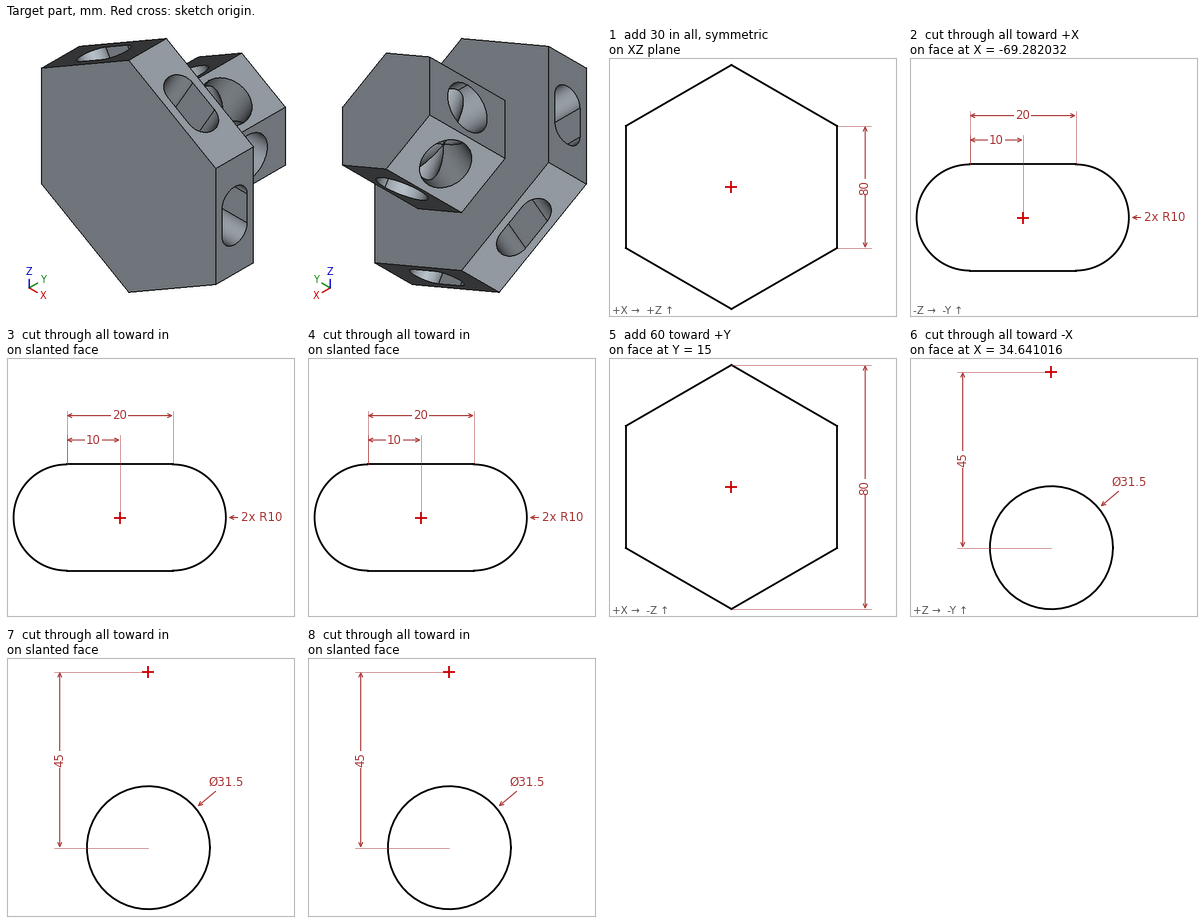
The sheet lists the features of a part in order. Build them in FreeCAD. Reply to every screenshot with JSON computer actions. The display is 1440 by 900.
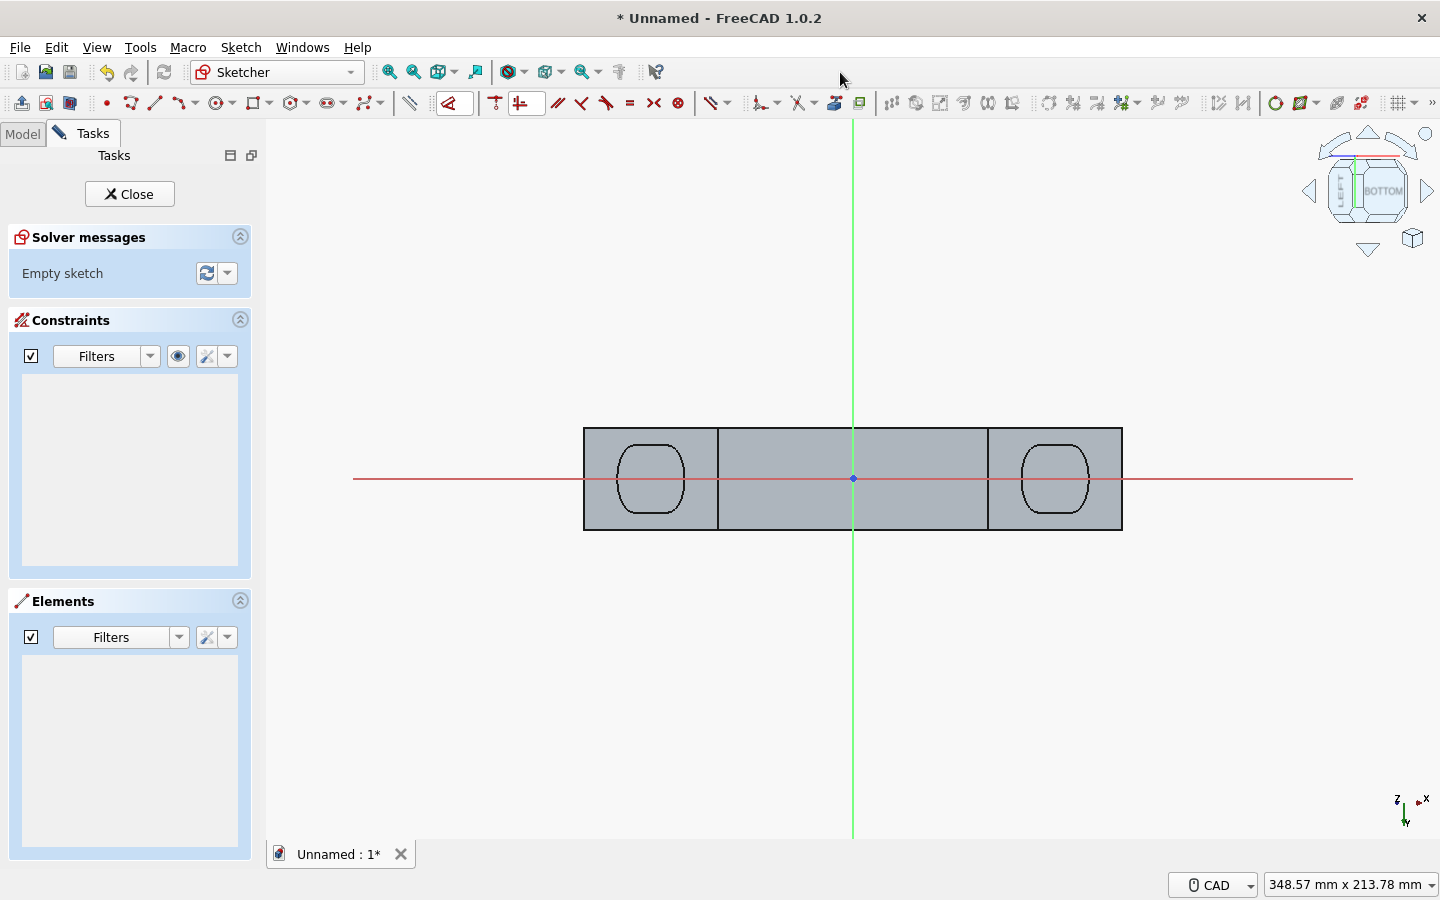
{"action": "left_click", "coordinate": [70, 104]}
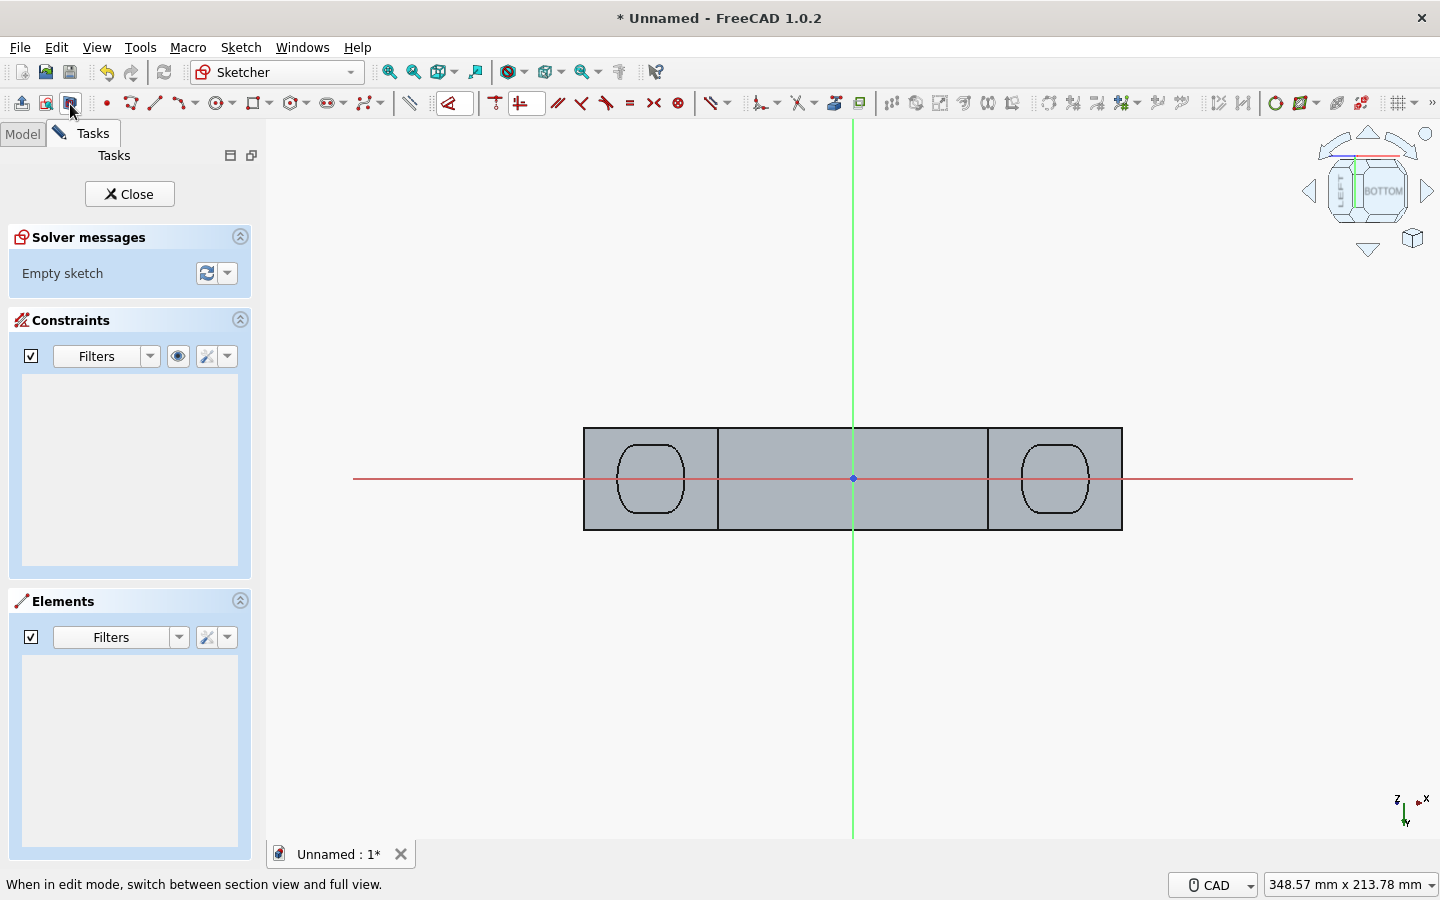
{"action": "scroll", "coordinate": [870, 479], "scroll_direction": "up", "scroll_amount": 8}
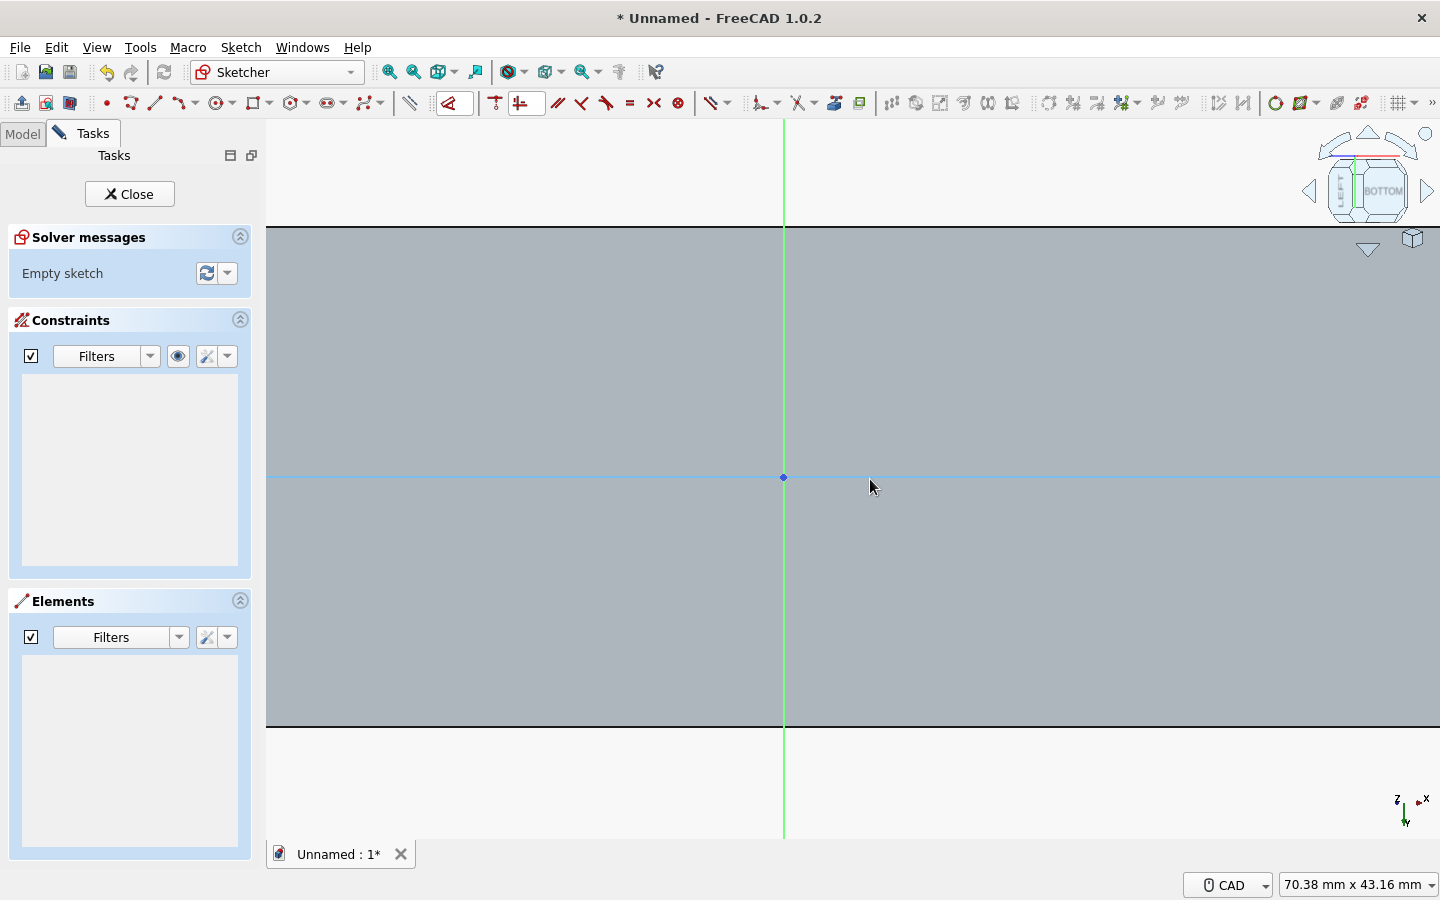
{"action": "left_click", "coordinate": [328, 104]}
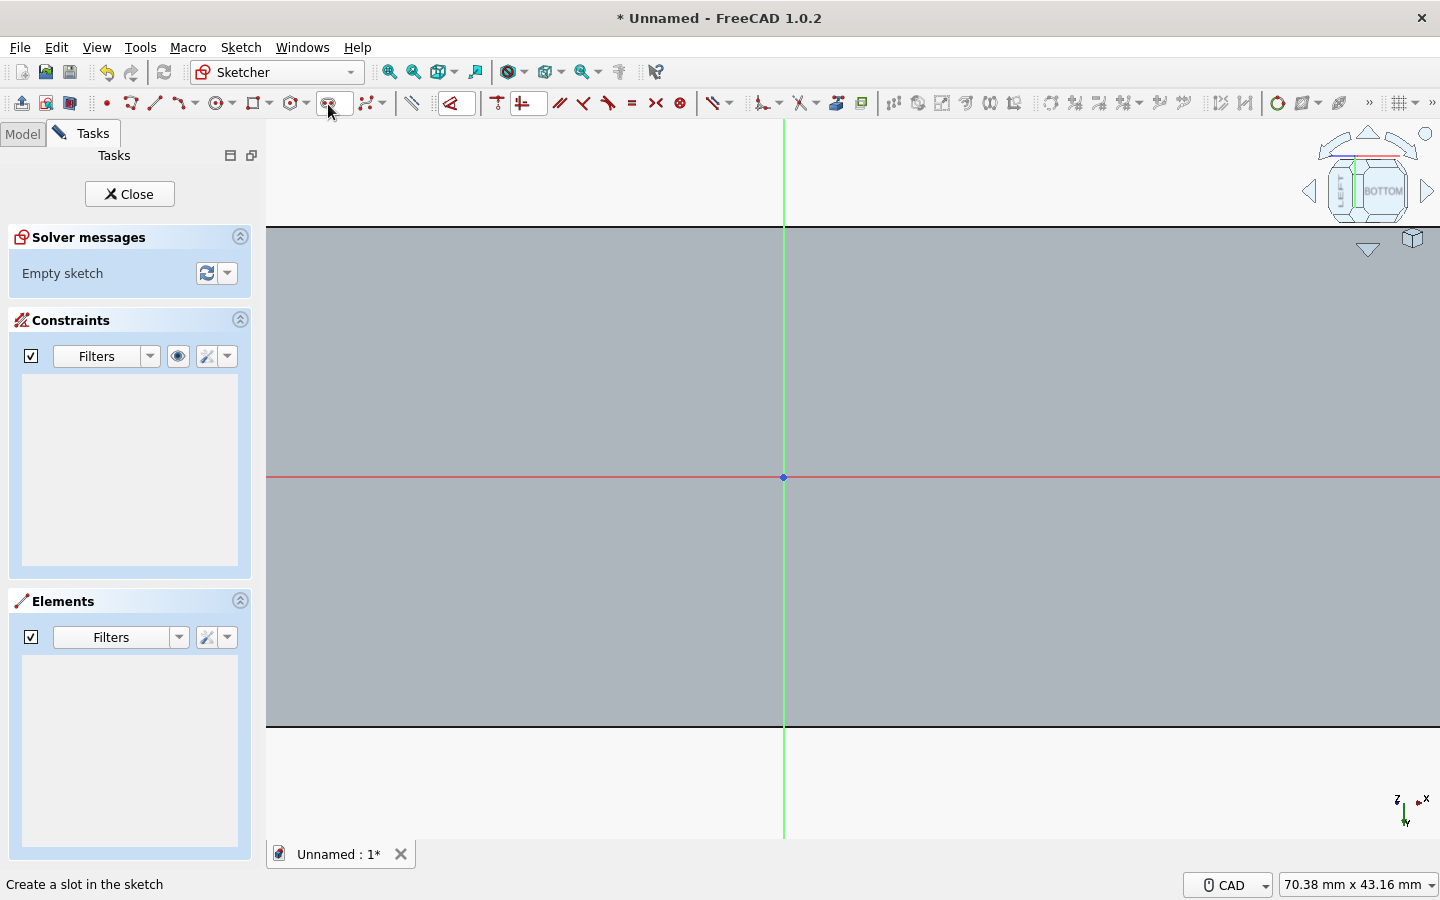
{"action": "left_click", "coordinate": [617, 477]}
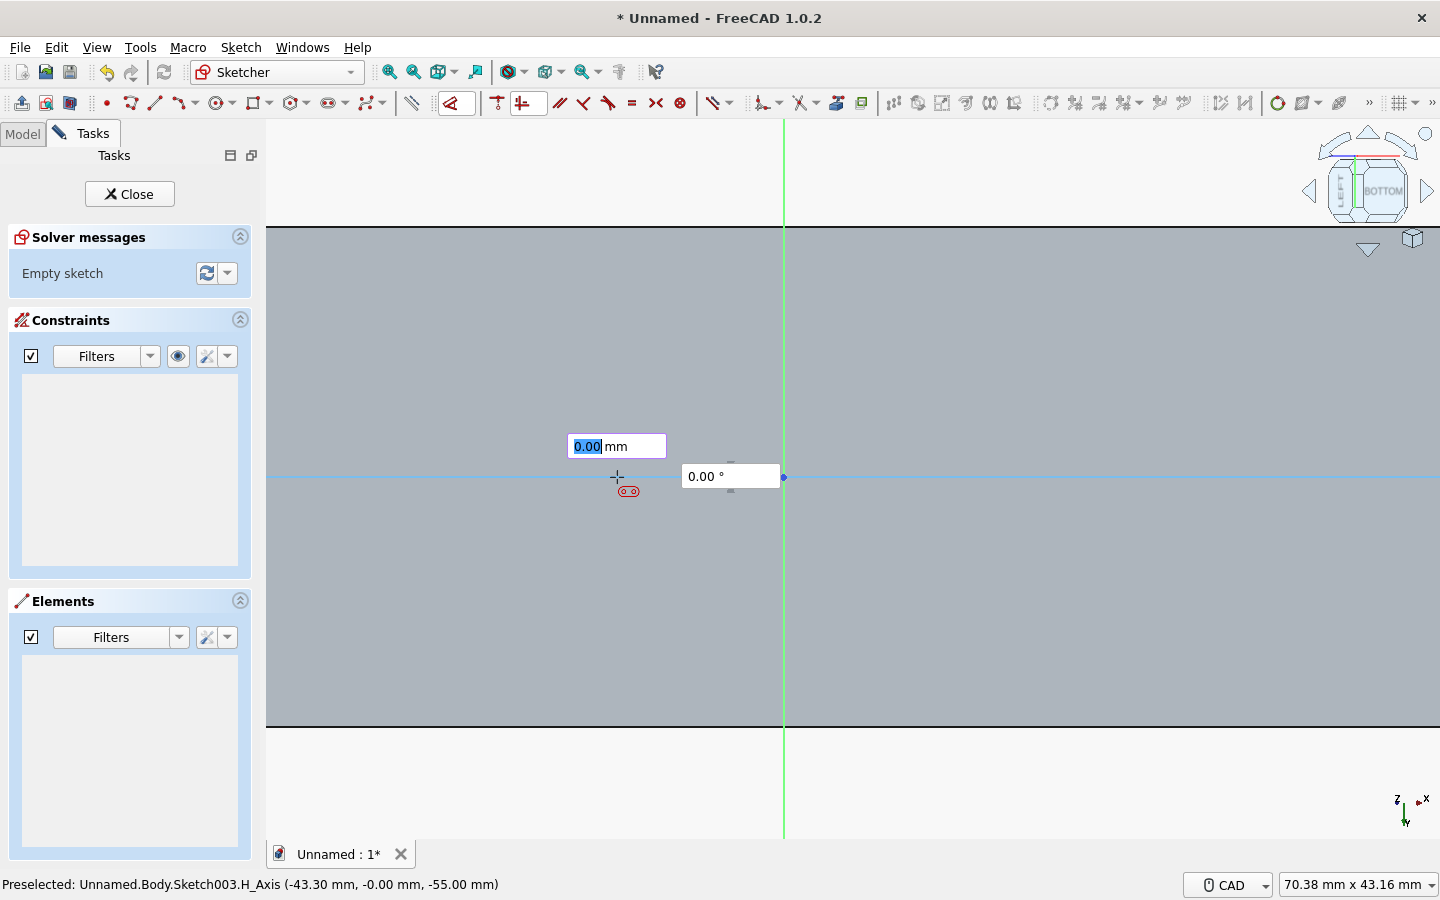
{"action": "left_click", "coordinate": [951, 468]}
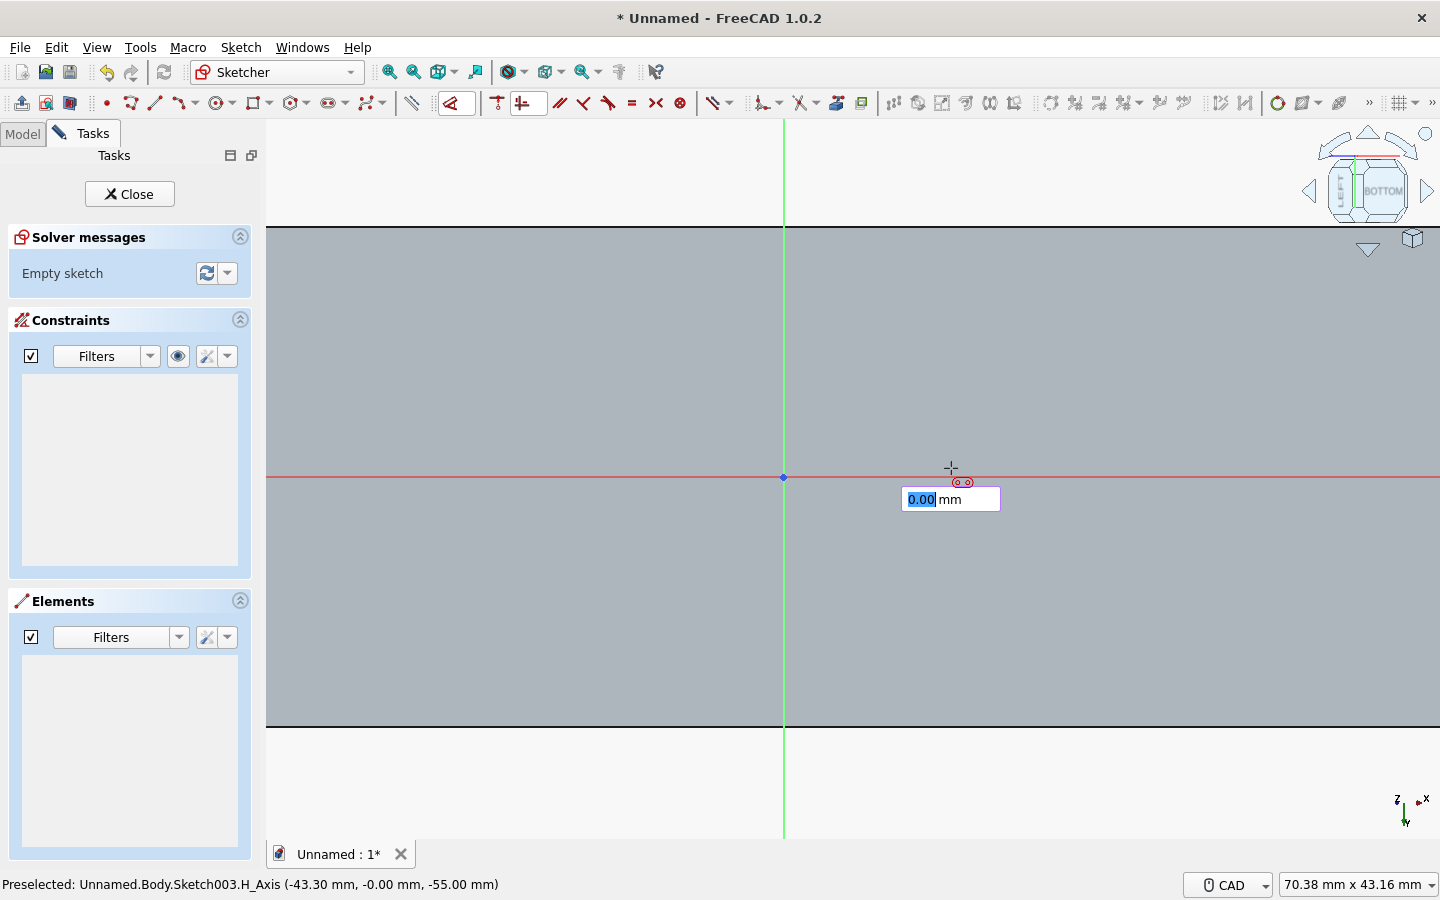
{"action": "left_click", "coordinate": [734, 644]}
{"action": "key", "text": "Escape"}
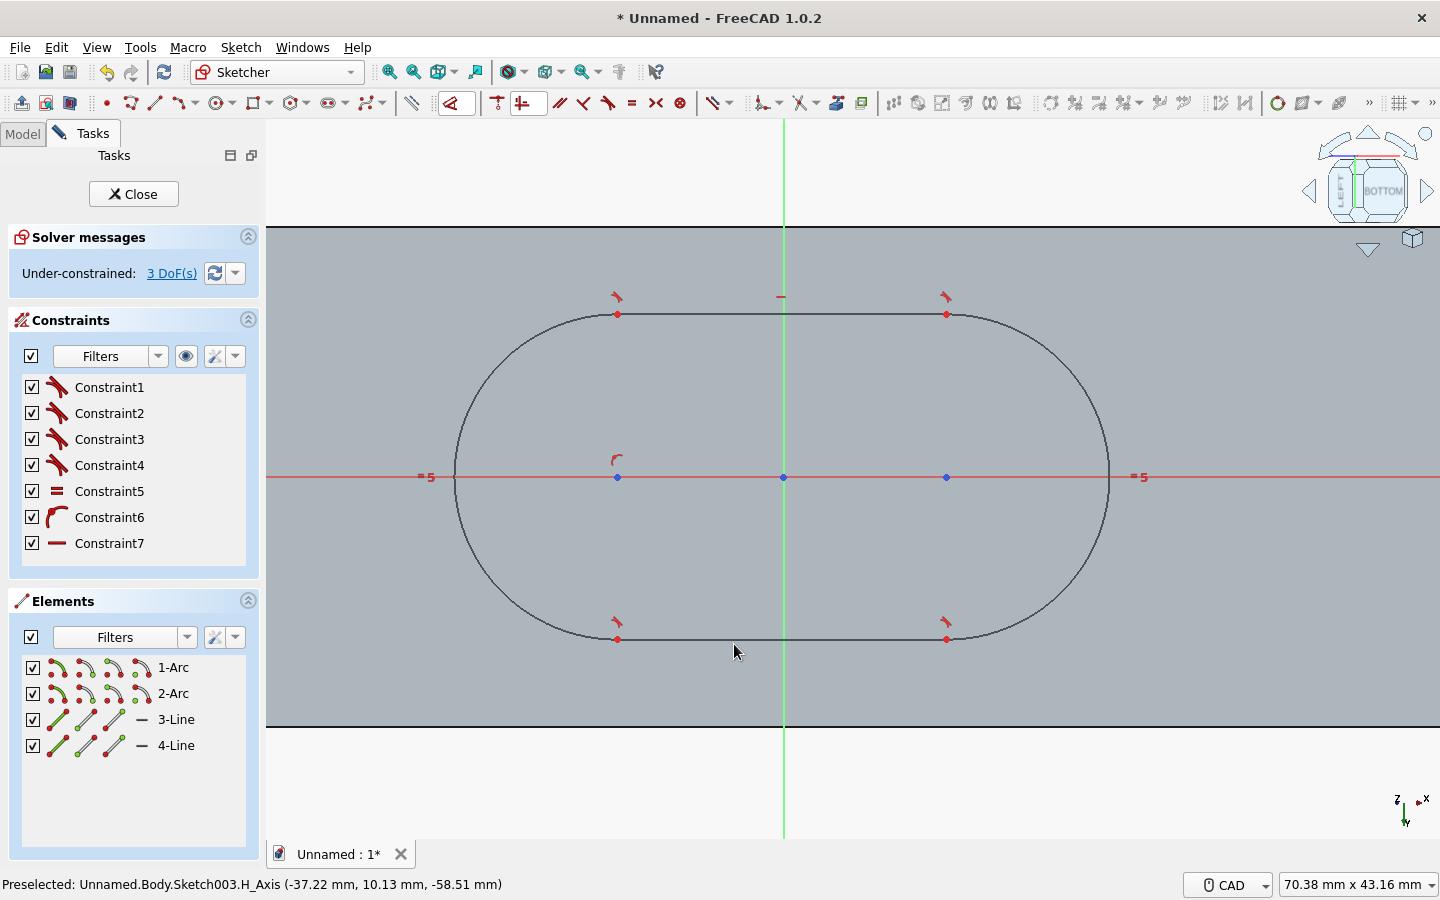
{"action": "left_click", "coordinate": [486, 381]}